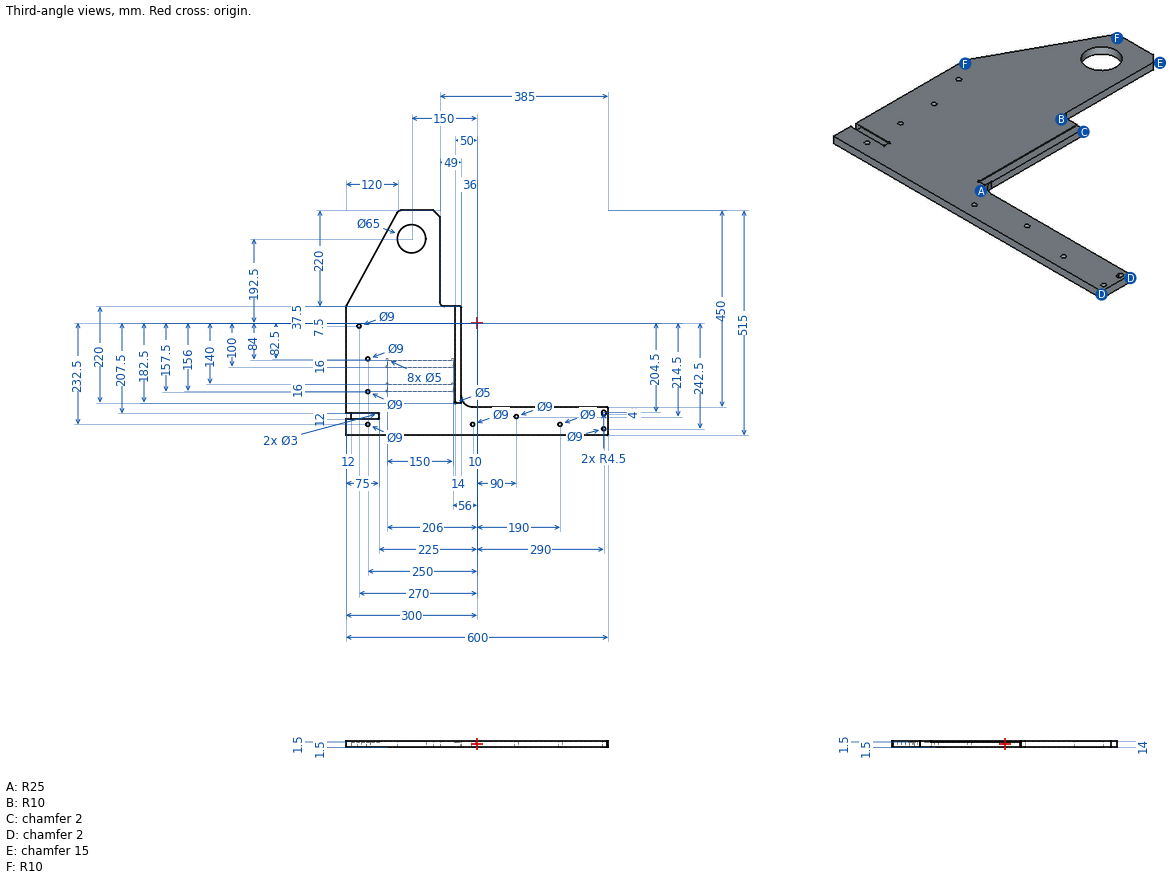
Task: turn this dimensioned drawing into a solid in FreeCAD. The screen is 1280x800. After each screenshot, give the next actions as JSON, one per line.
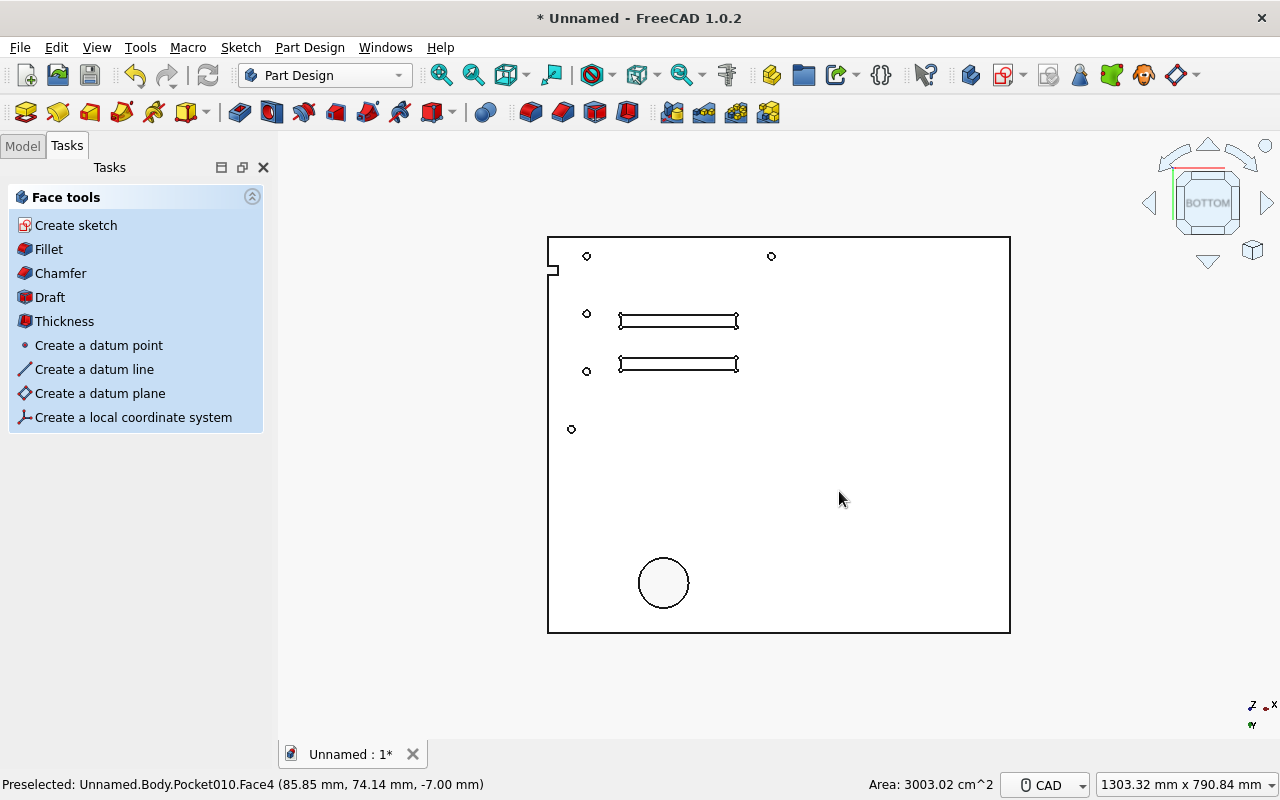
{"action": "left_click", "coordinate": [1004, 76]}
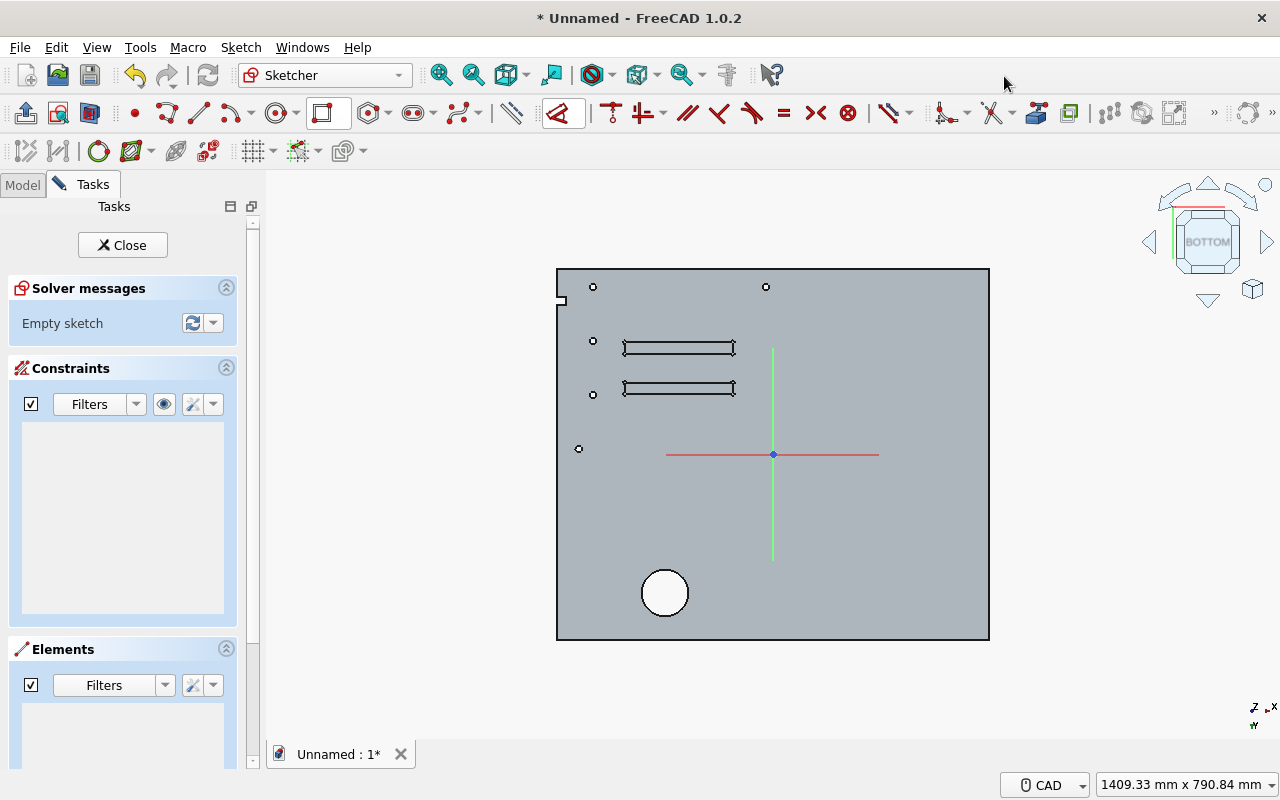
{"action": "scroll", "coordinate": [845, 292], "scroll_direction": "up", "scroll_amount": 15}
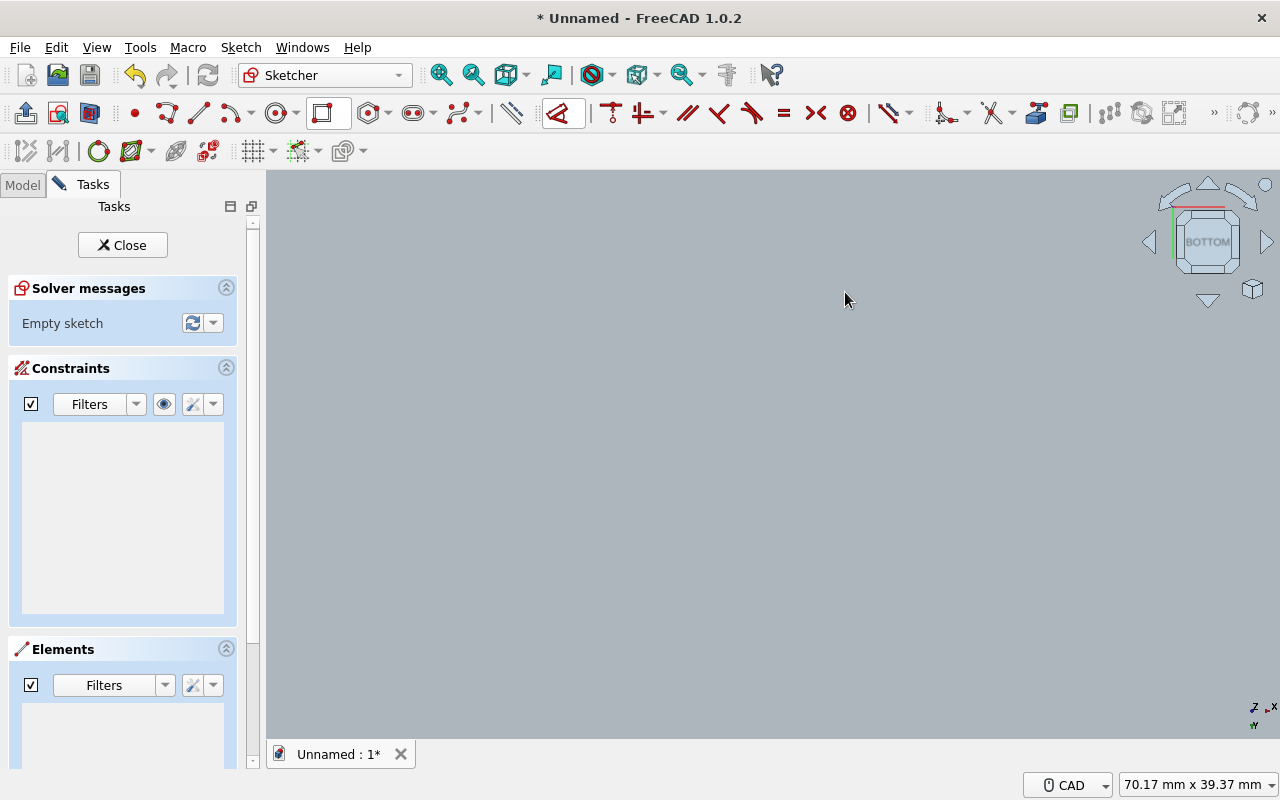
{"action": "scroll", "coordinate": [679, 451], "scroll_direction": "up", "scroll_amount": 5}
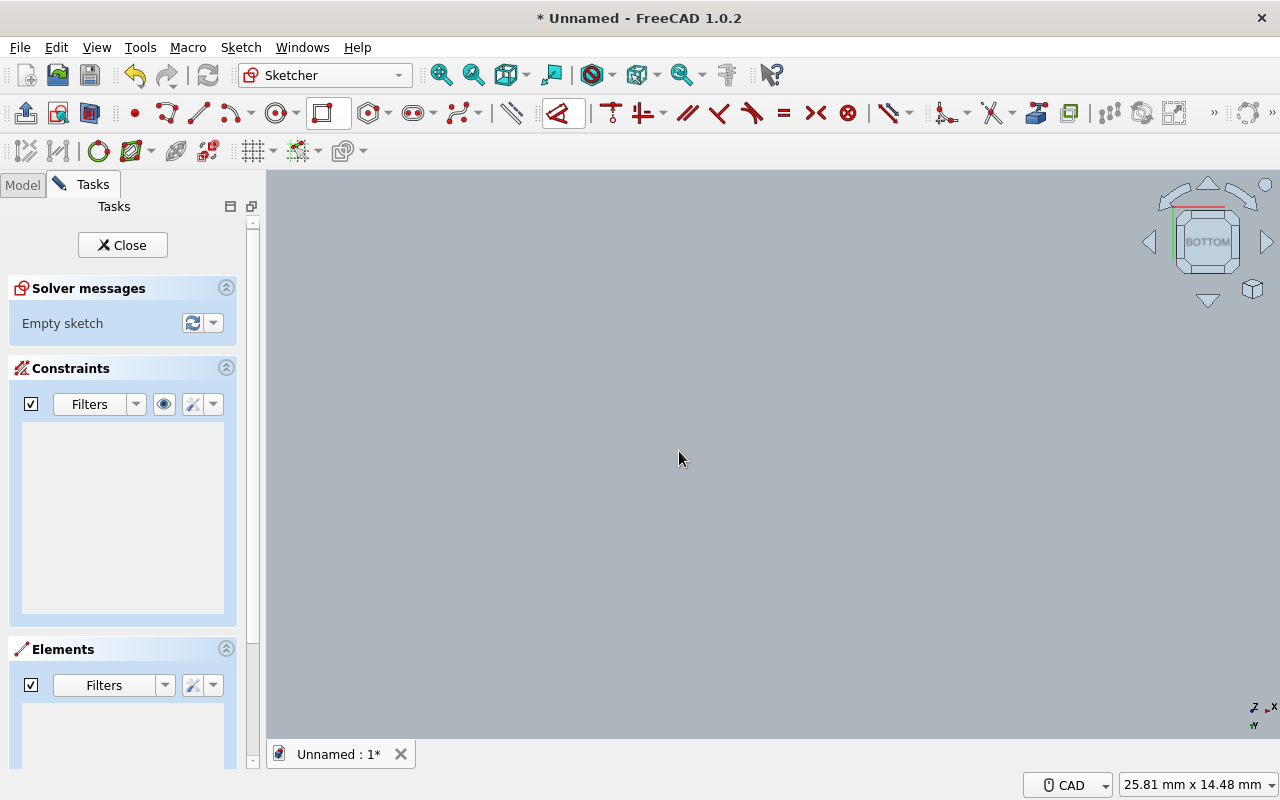
{"action": "left_click", "coordinate": [276, 114]}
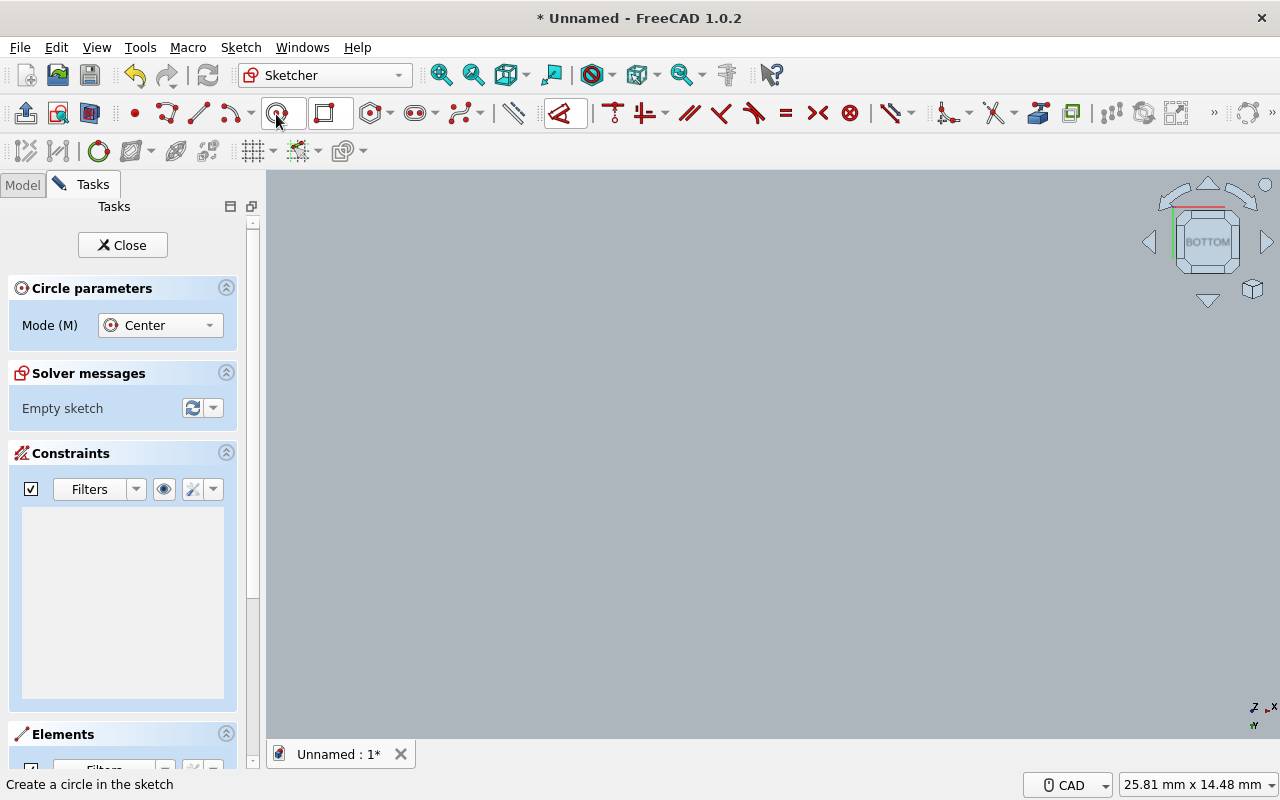
{"action": "left_click", "coordinate": [704, 453]}
{"action": "mouse_move", "coordinate": [829, 328]}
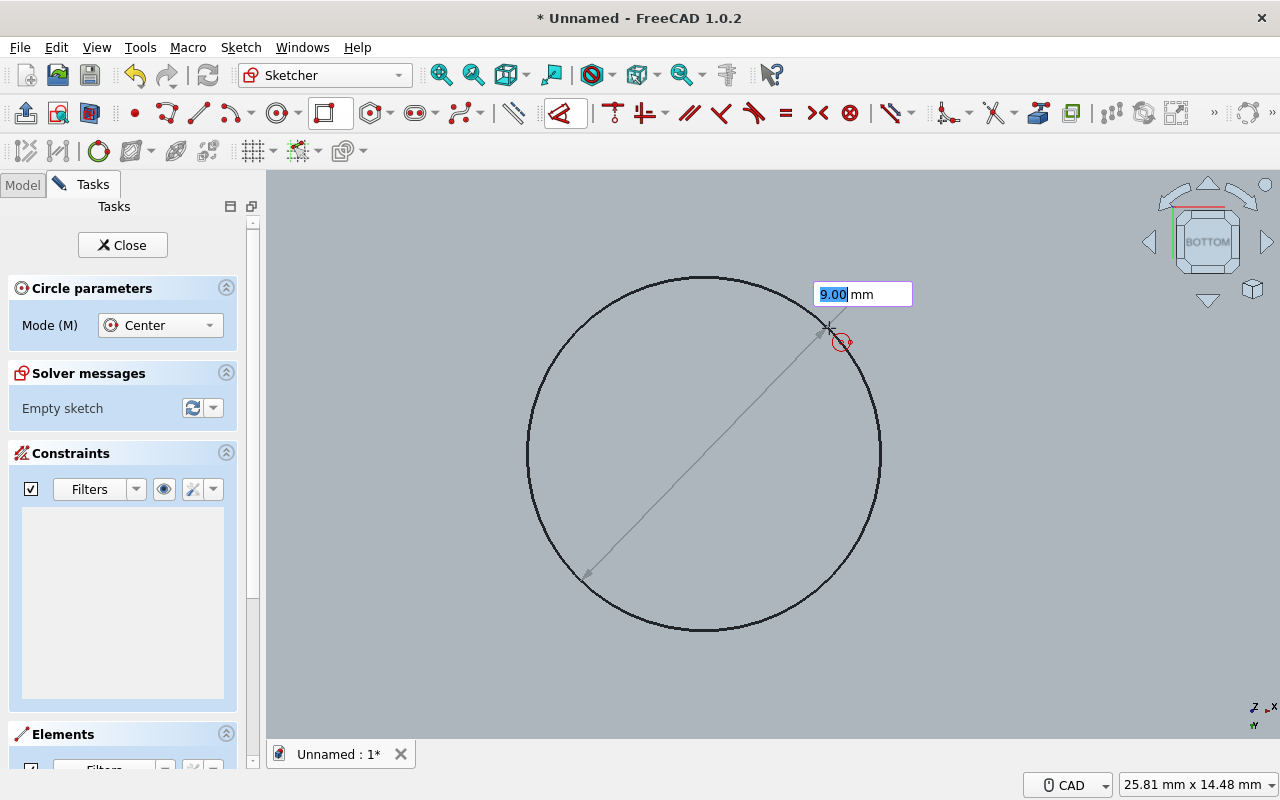
{"action": "type", "text": "9"}
{"action": "key", "text": "Return"}
{"action": "key", "text": "Escape"}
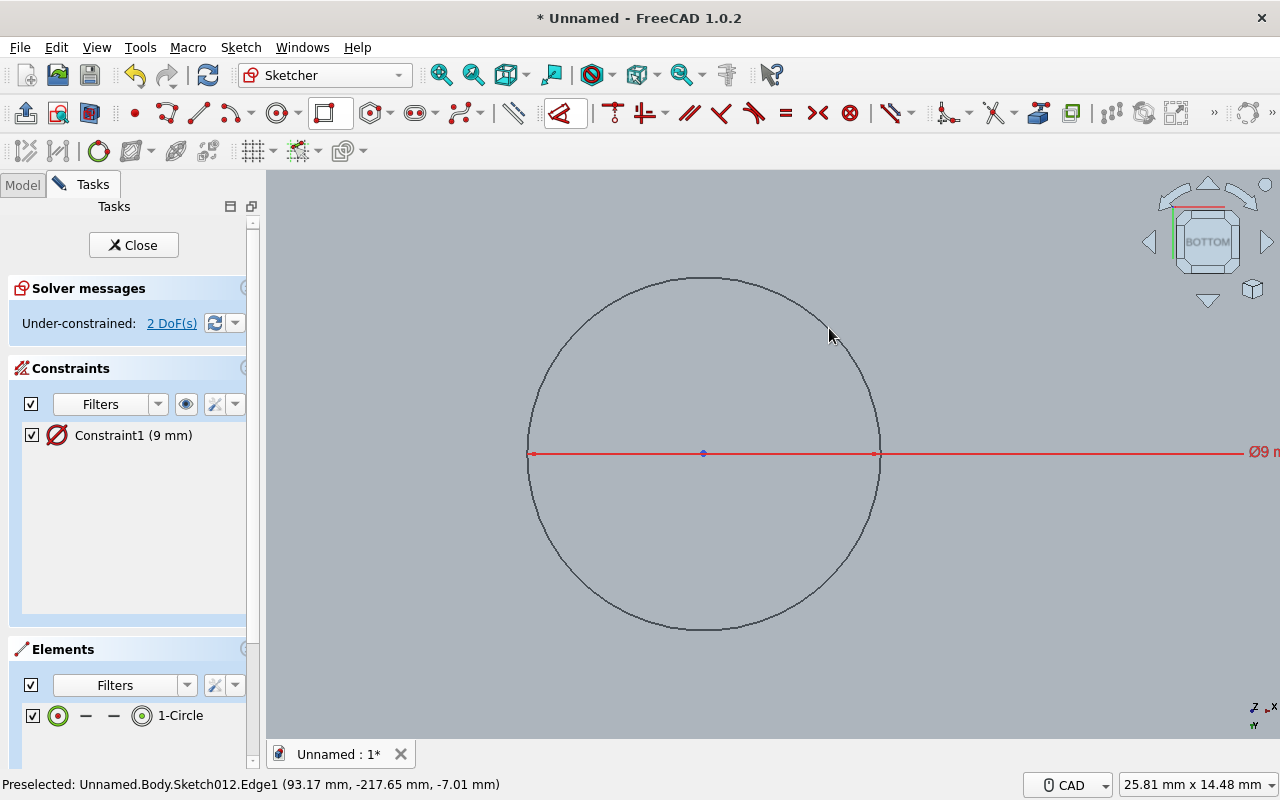
{"action": "left_click", "coordinate": [704, 454]}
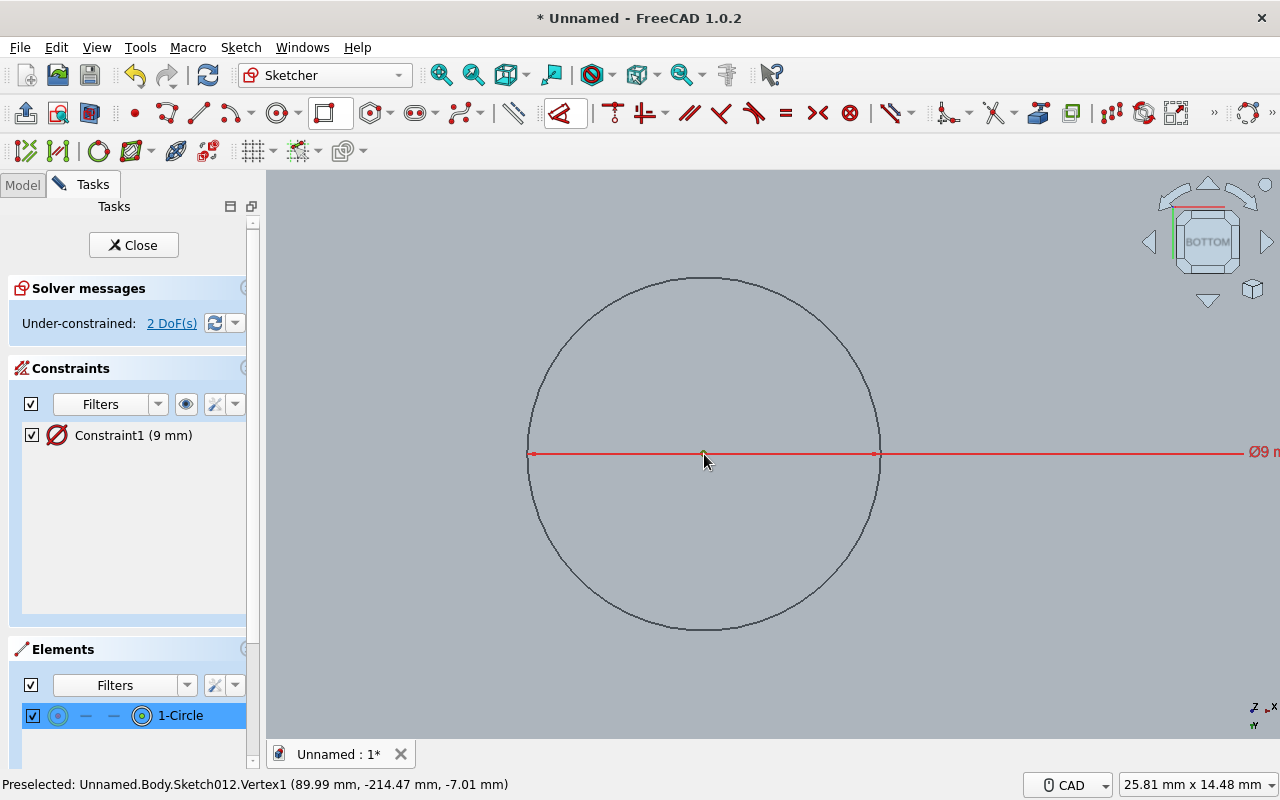
{"action": "left_click", "coordinate": [582, 114]}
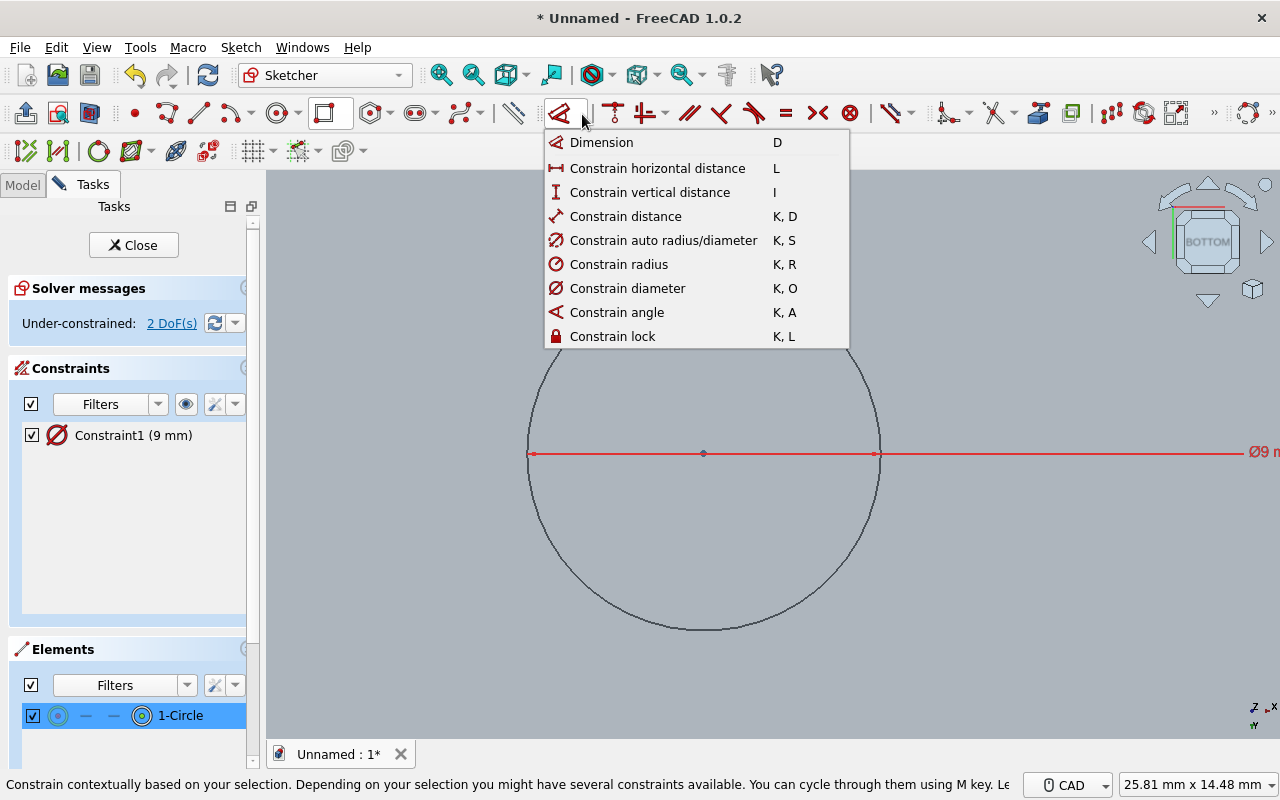
{"action": "left_click", "coordinate": [697, 168]}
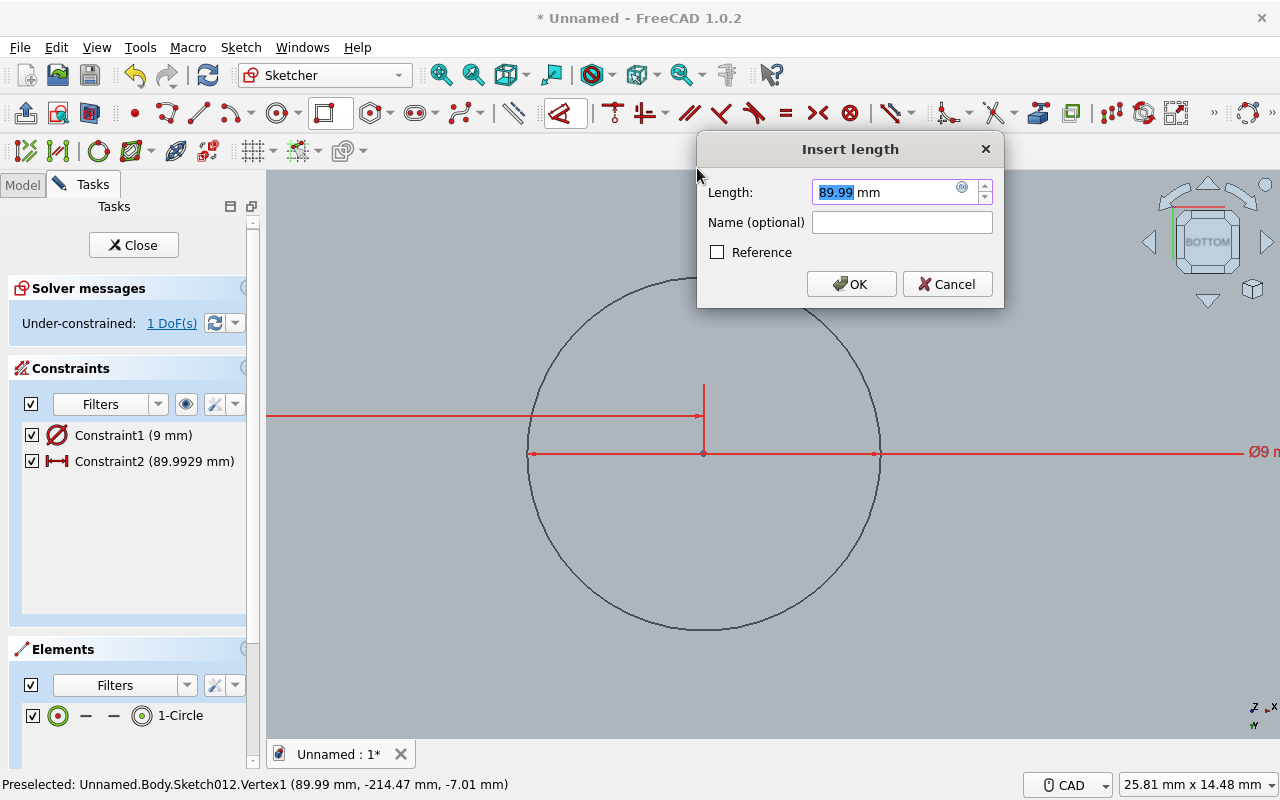
{"action": "type", "text": "90"}
{"action": "key", "text": "Return"}